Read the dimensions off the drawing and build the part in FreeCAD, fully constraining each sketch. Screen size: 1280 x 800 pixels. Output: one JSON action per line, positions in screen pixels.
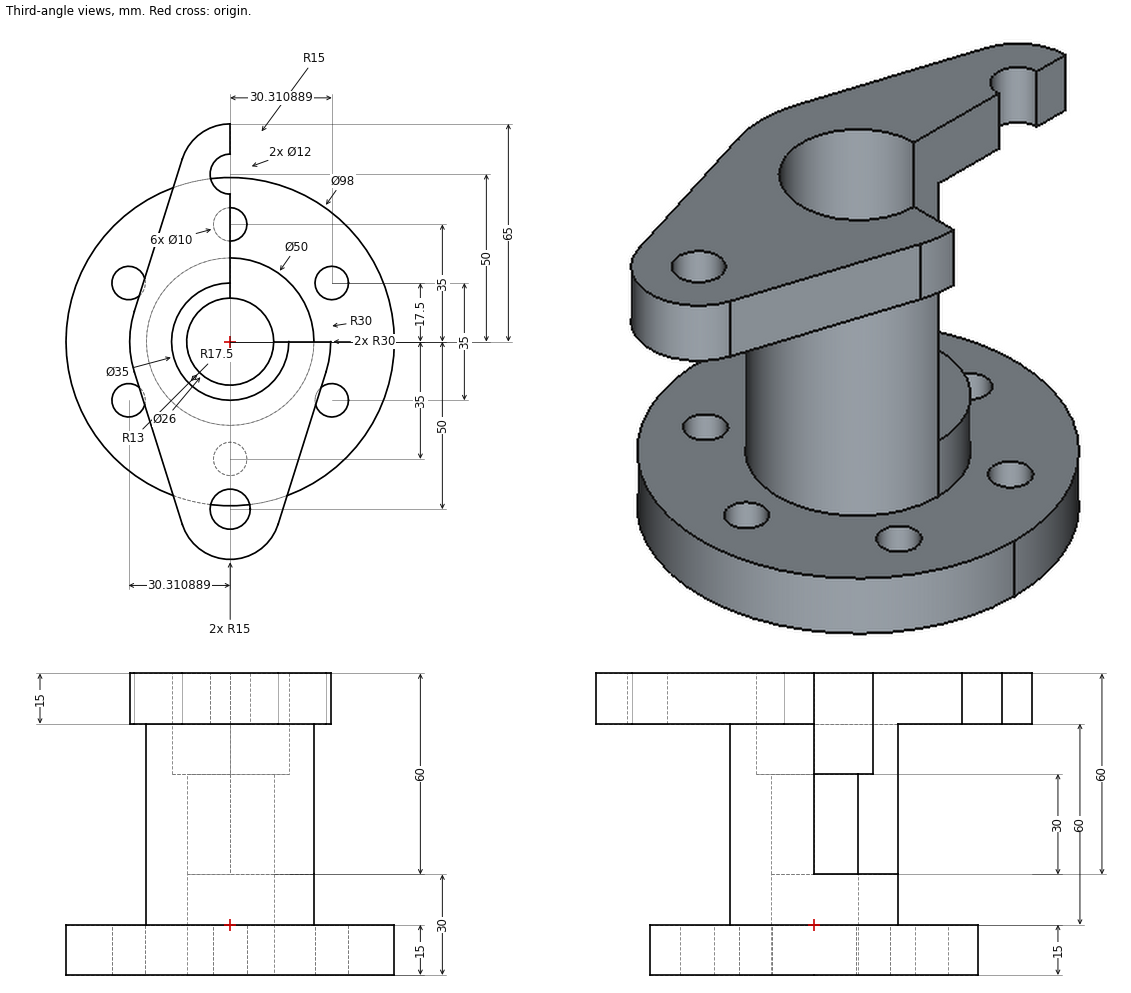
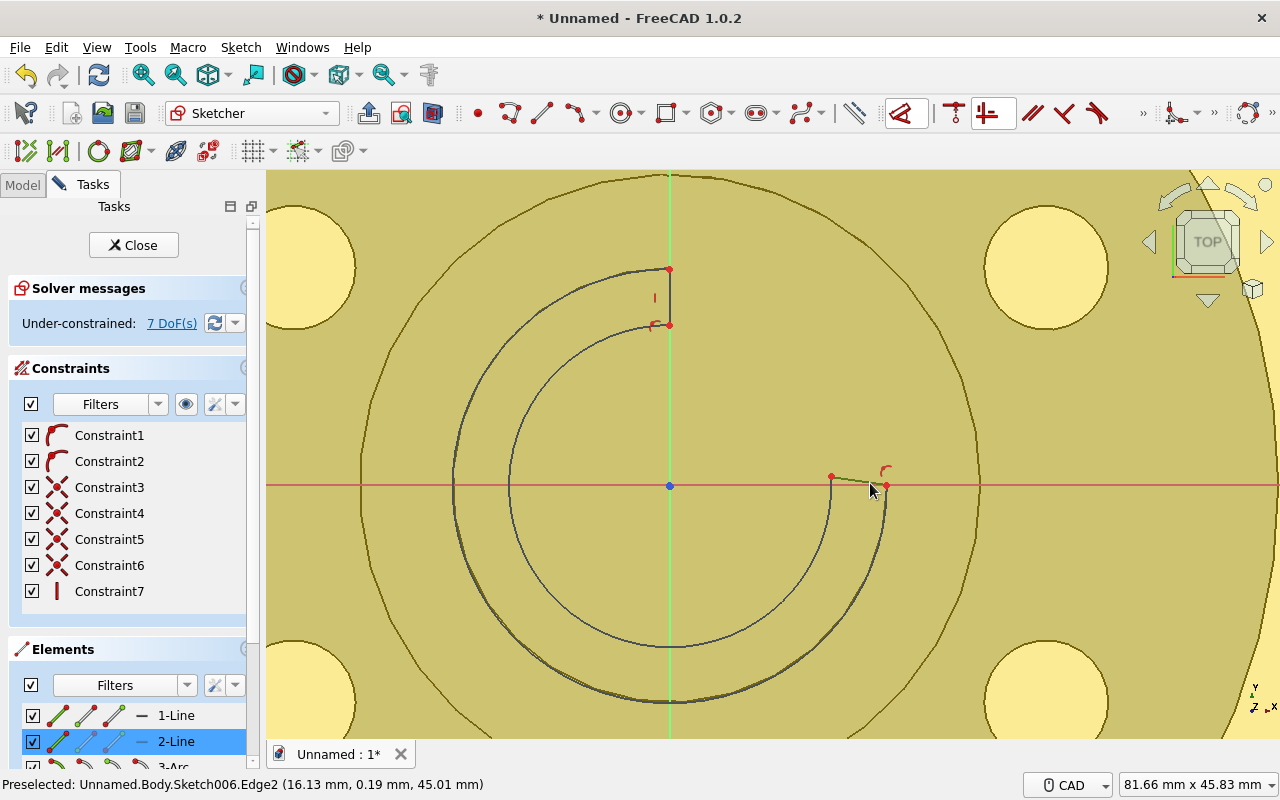
{"action": "key", "text": "h"}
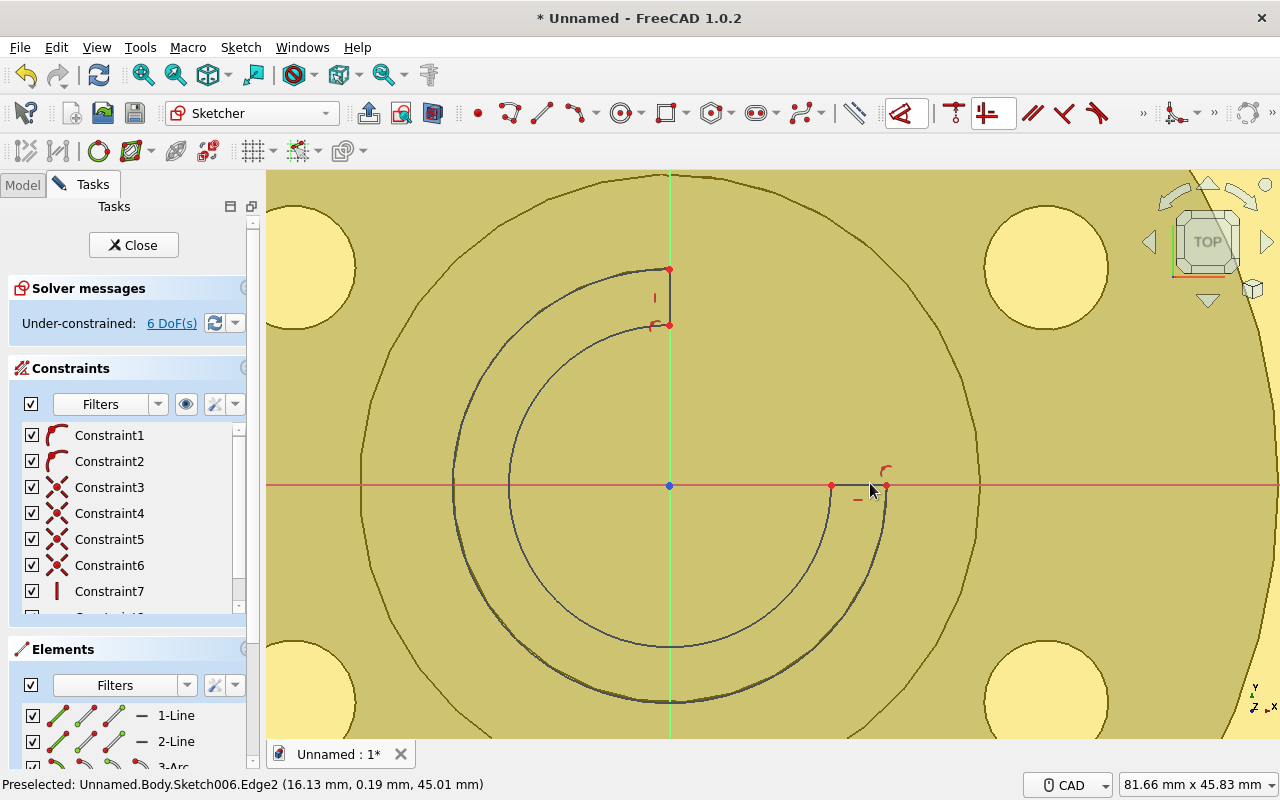
{"action": "left_click", "coordinate": [455, 452]}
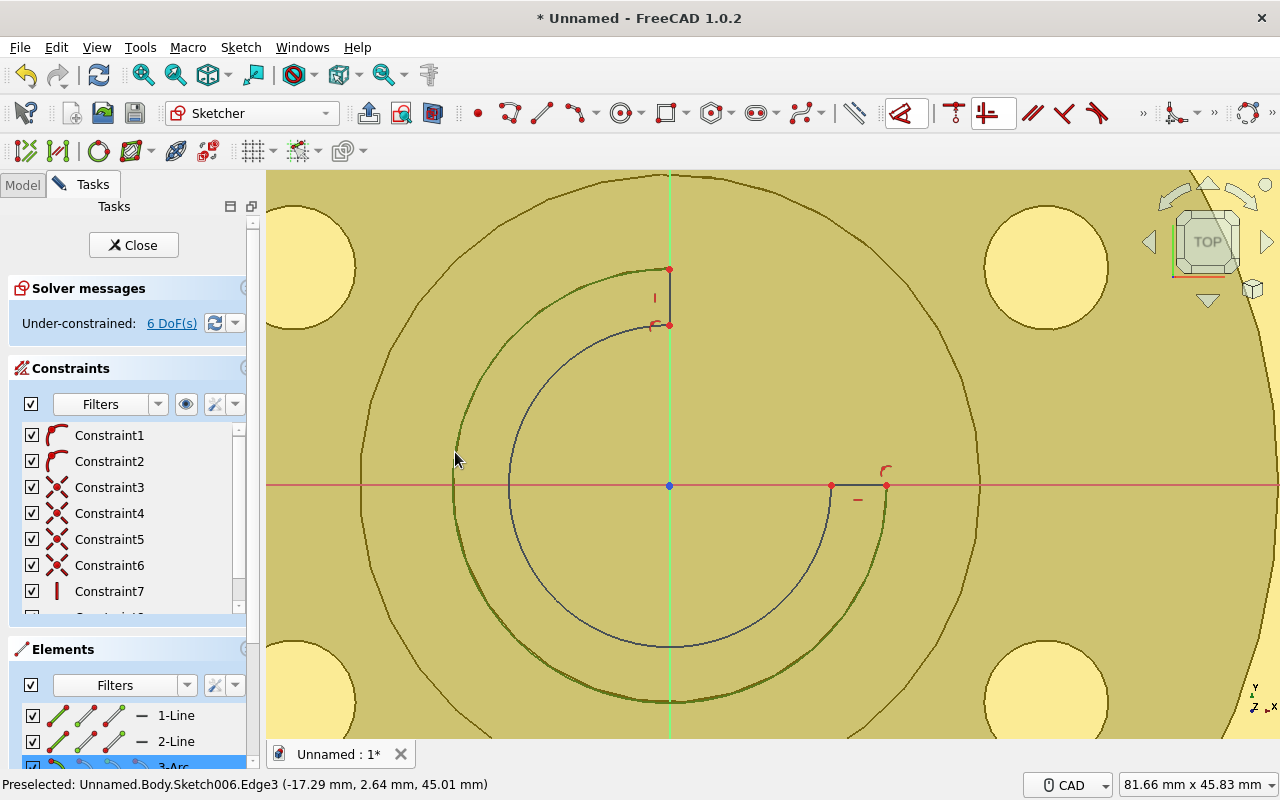
{"action": "left_click", "coordinate": [511, 461]}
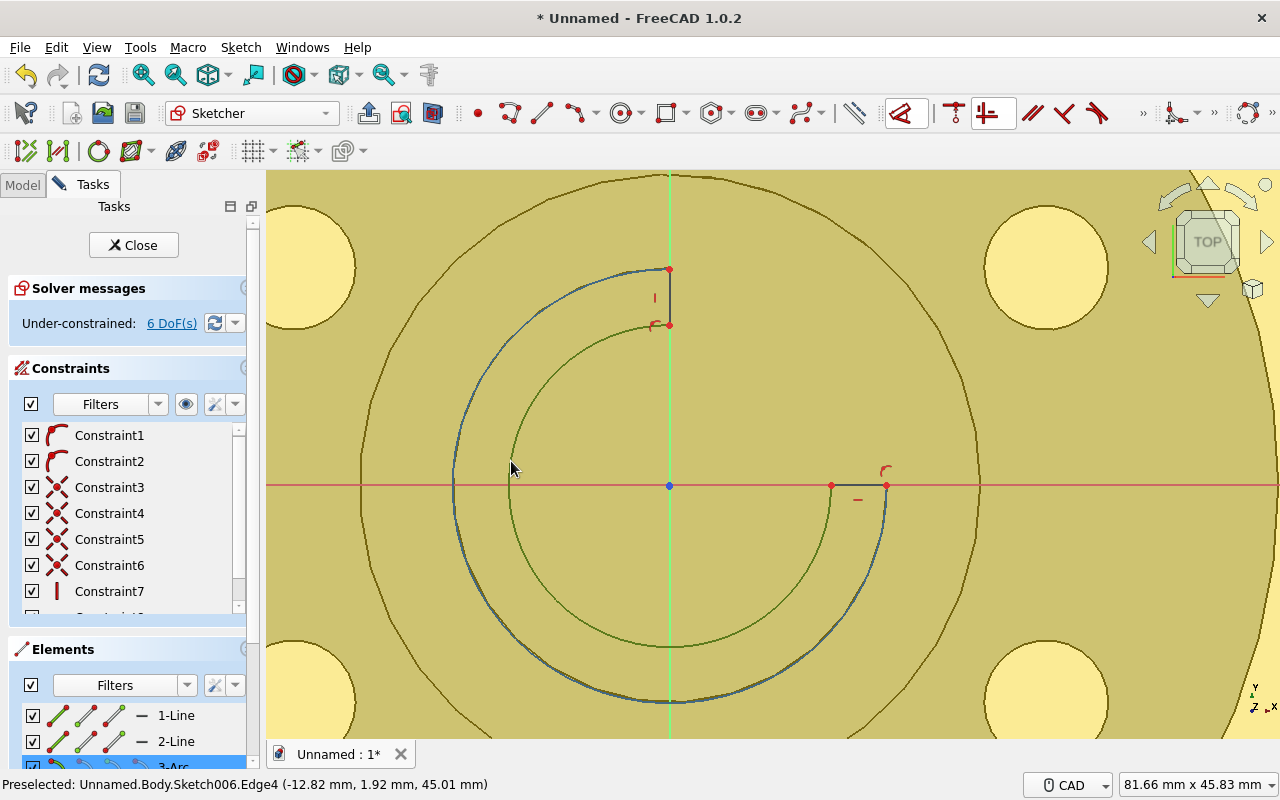
{"action": "key", "text": "c"}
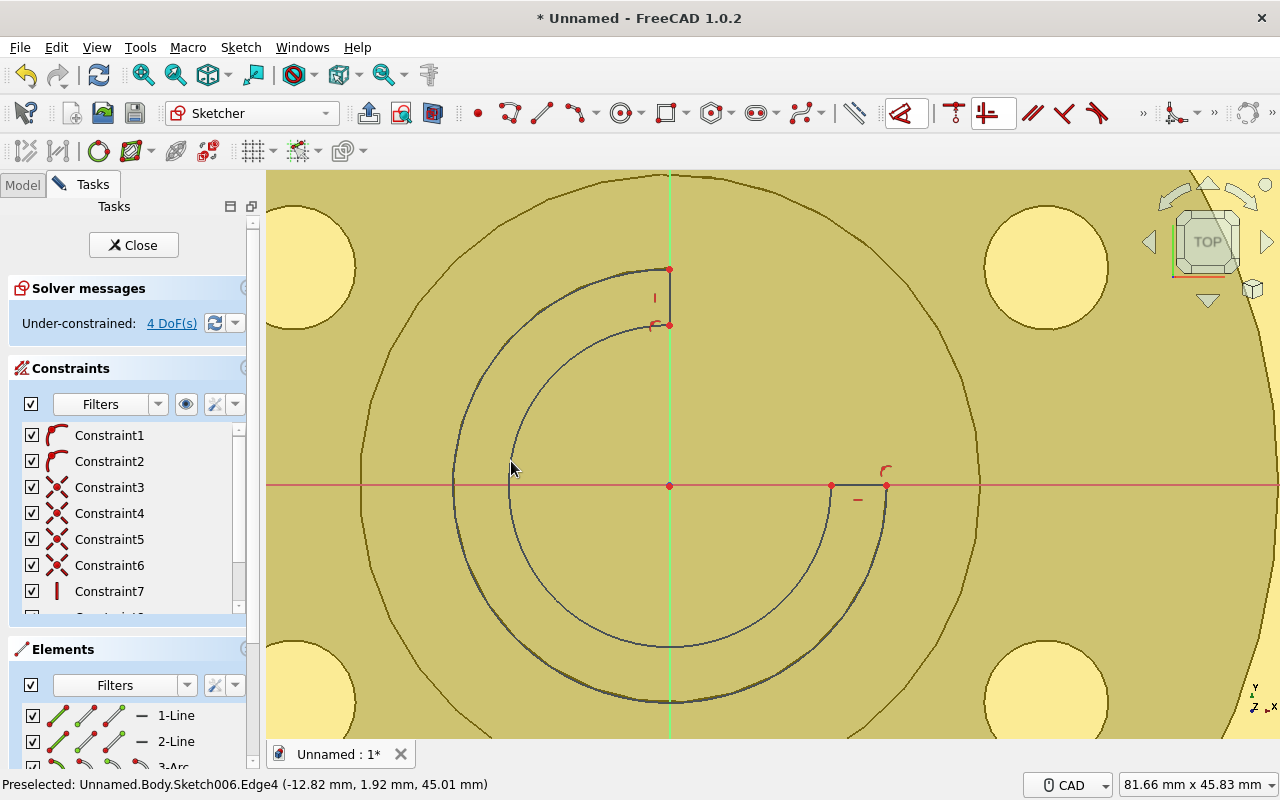
{"action": "left_click_drag", "start_coordinate": [660, 475], "coordinate": [680, 496]}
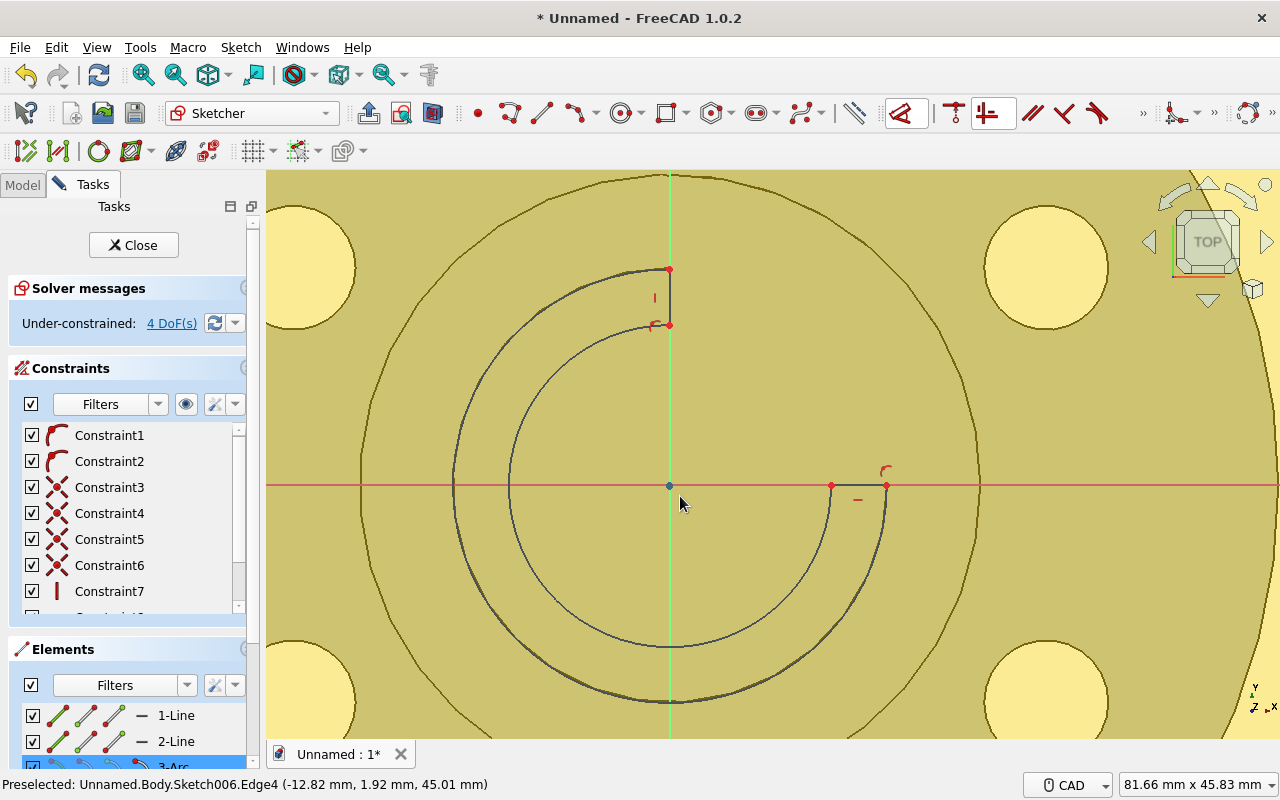
{"action": "left_click", "coordinate": [954, 114]}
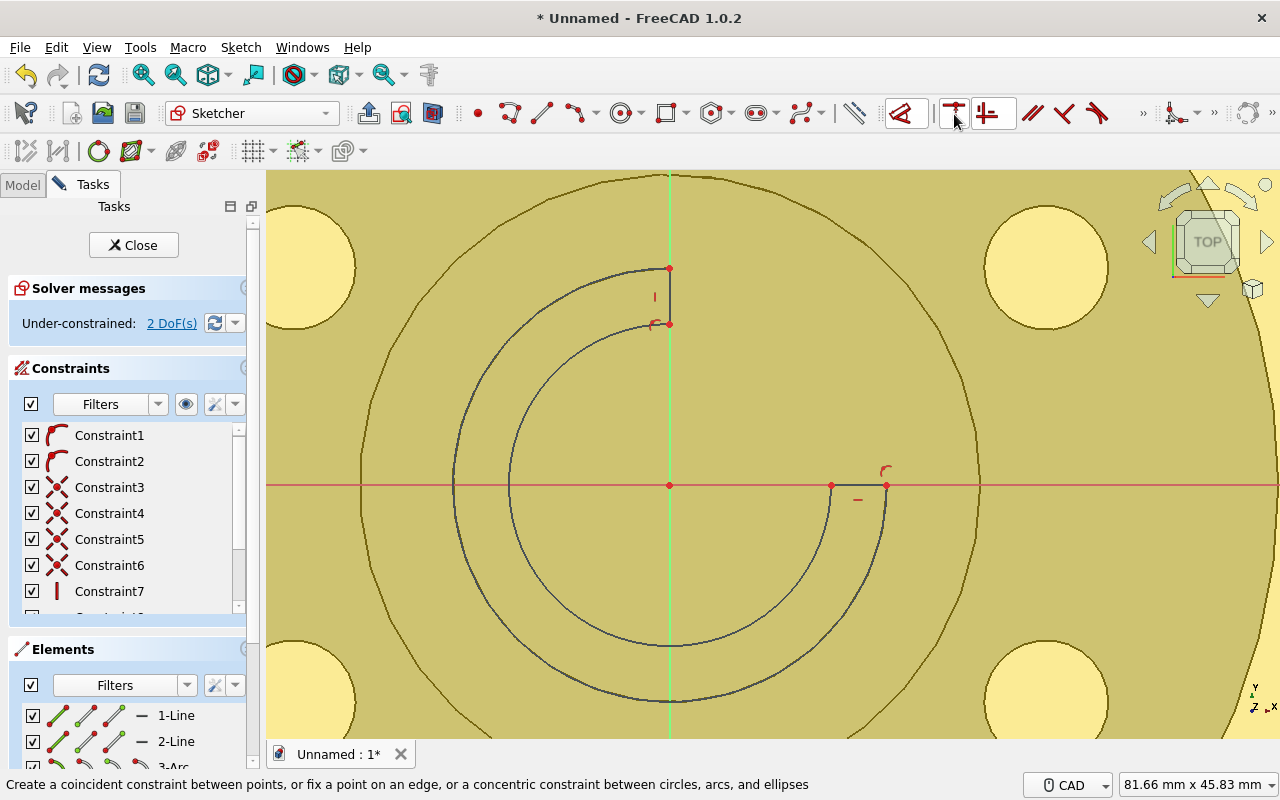
{"action": "left_click", "coordinate": [456, 451]}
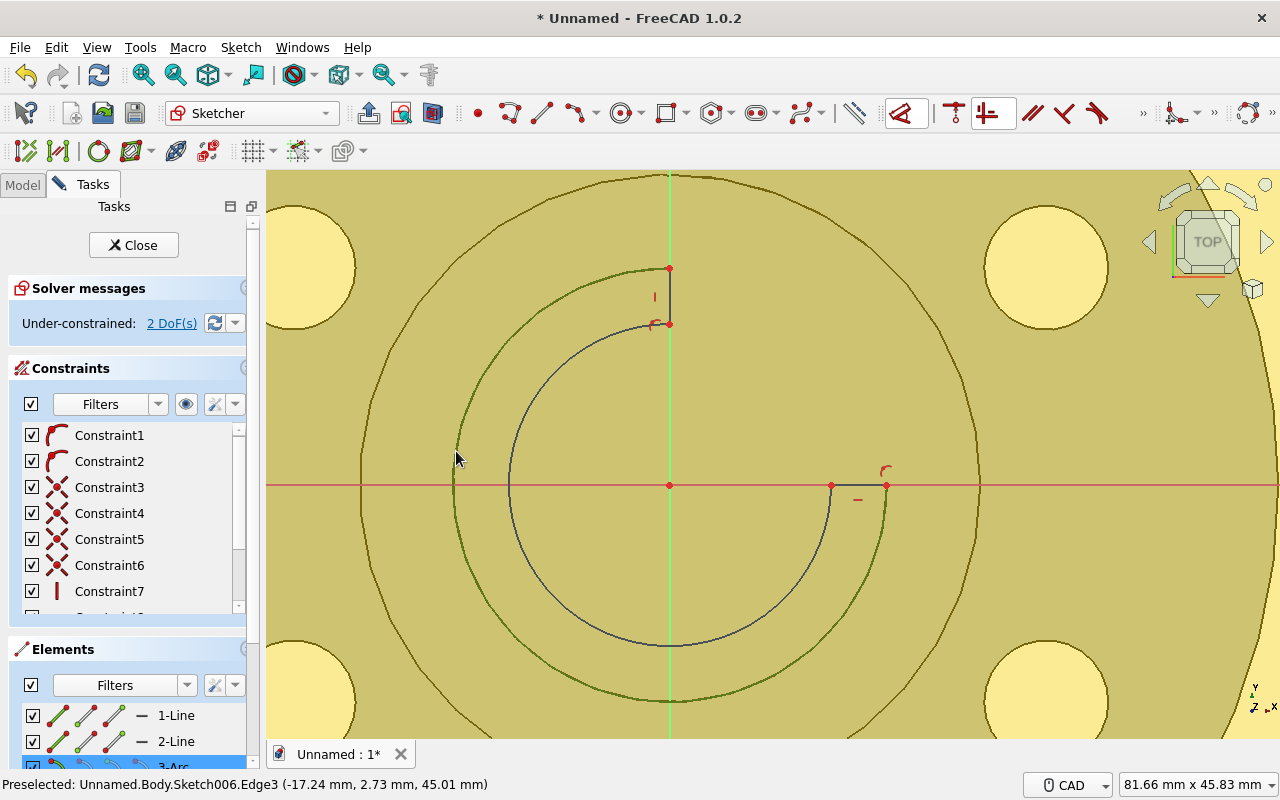
{"action": "left_click", "coordinate": [922, 114]}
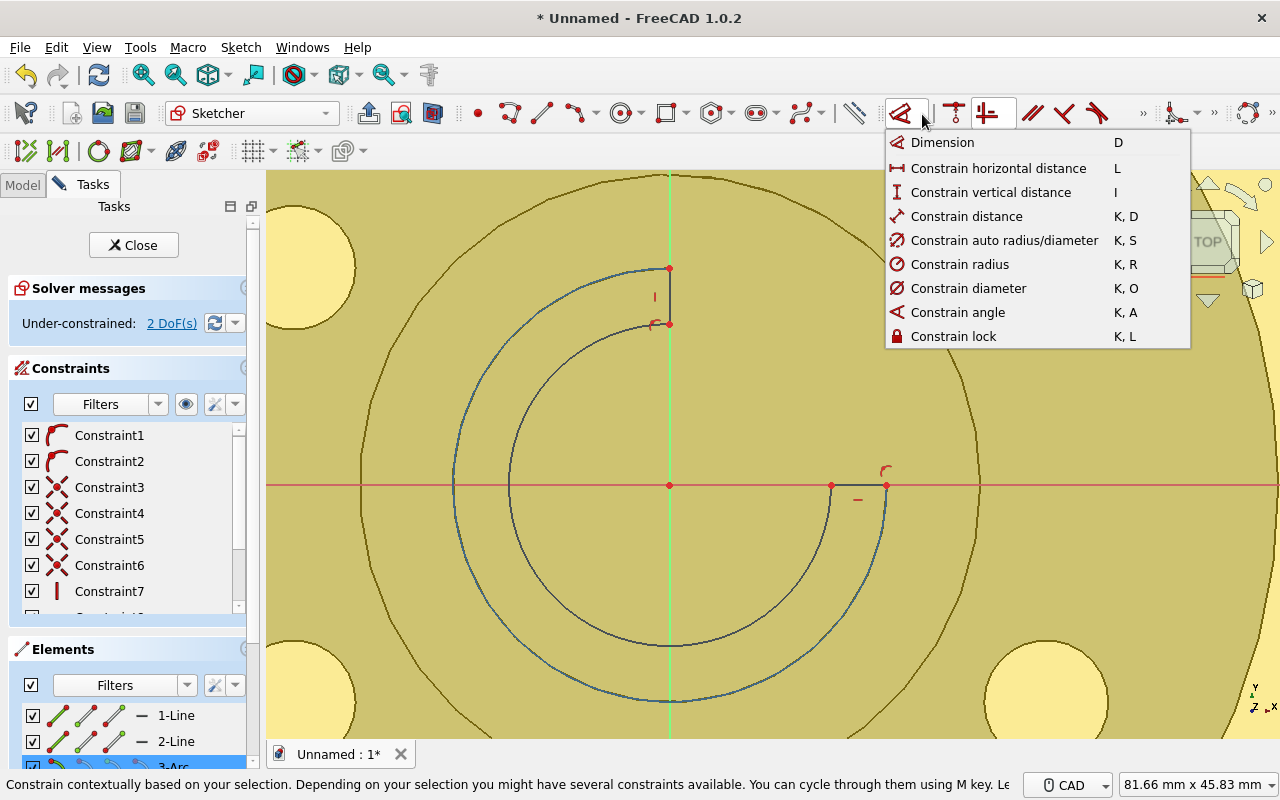
{"action": "left_click", "coordinate": [1038, 264]}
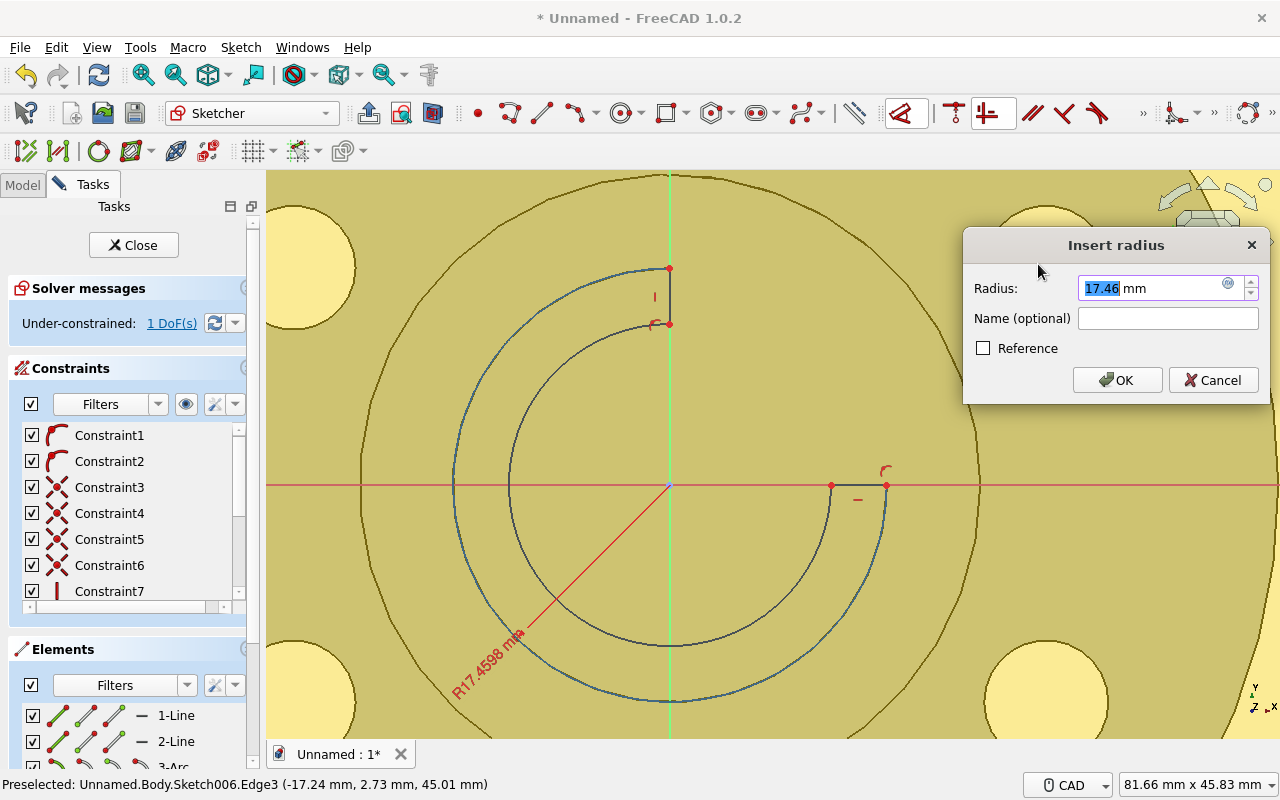
{"action": "type", "text": "17.5"}
{"action": "key", "text": "Return"}